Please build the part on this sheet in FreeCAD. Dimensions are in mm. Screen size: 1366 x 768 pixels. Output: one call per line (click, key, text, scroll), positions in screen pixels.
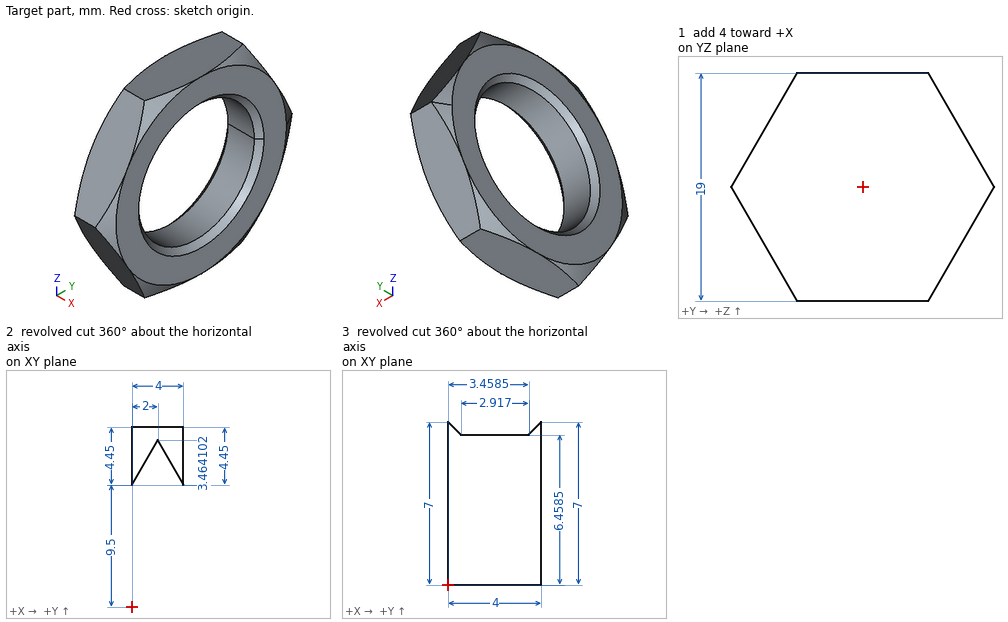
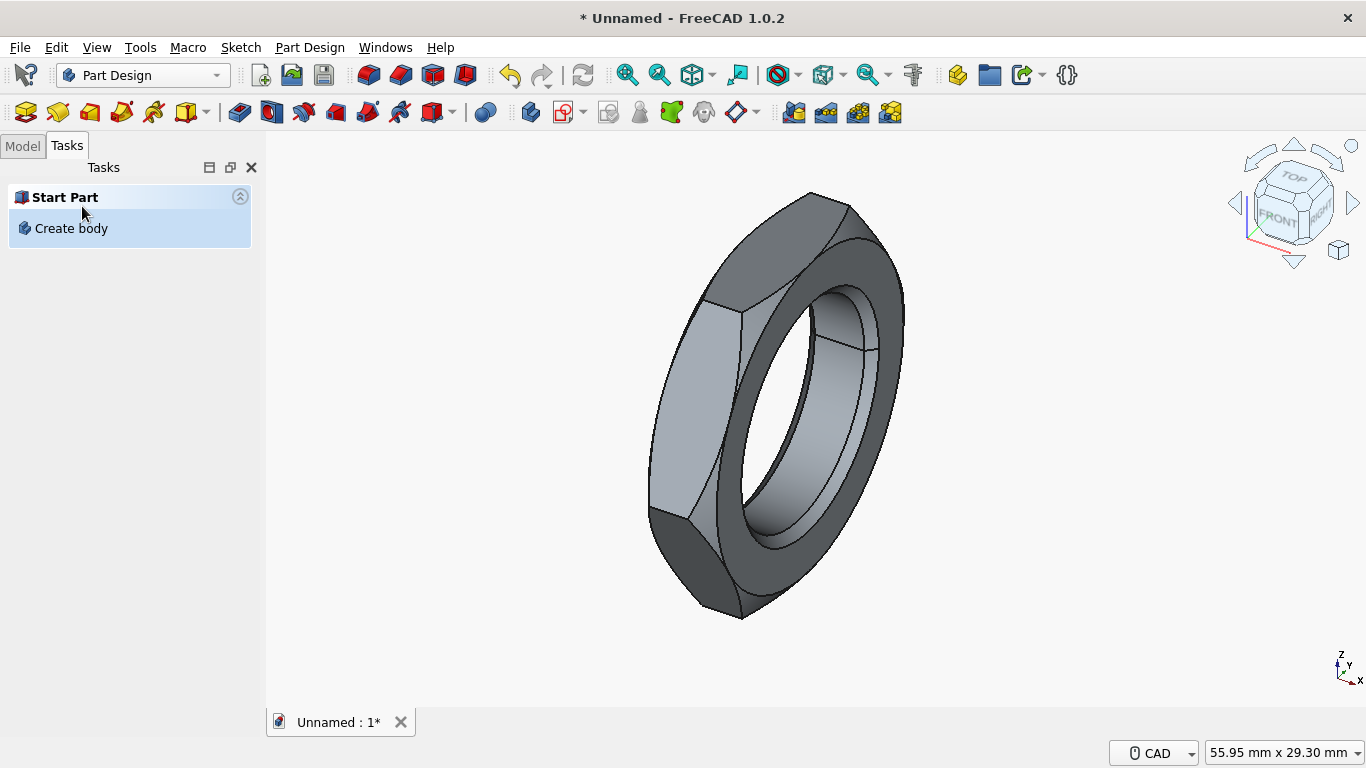
key(0)